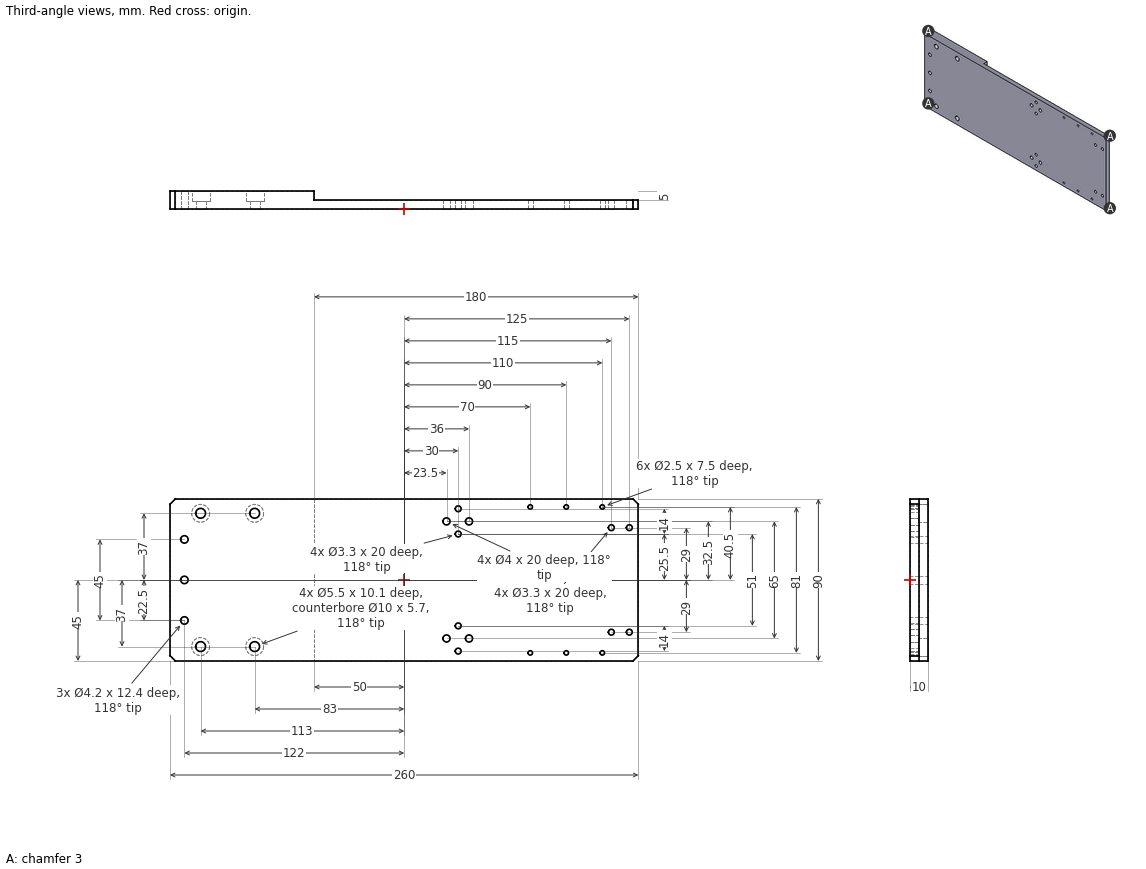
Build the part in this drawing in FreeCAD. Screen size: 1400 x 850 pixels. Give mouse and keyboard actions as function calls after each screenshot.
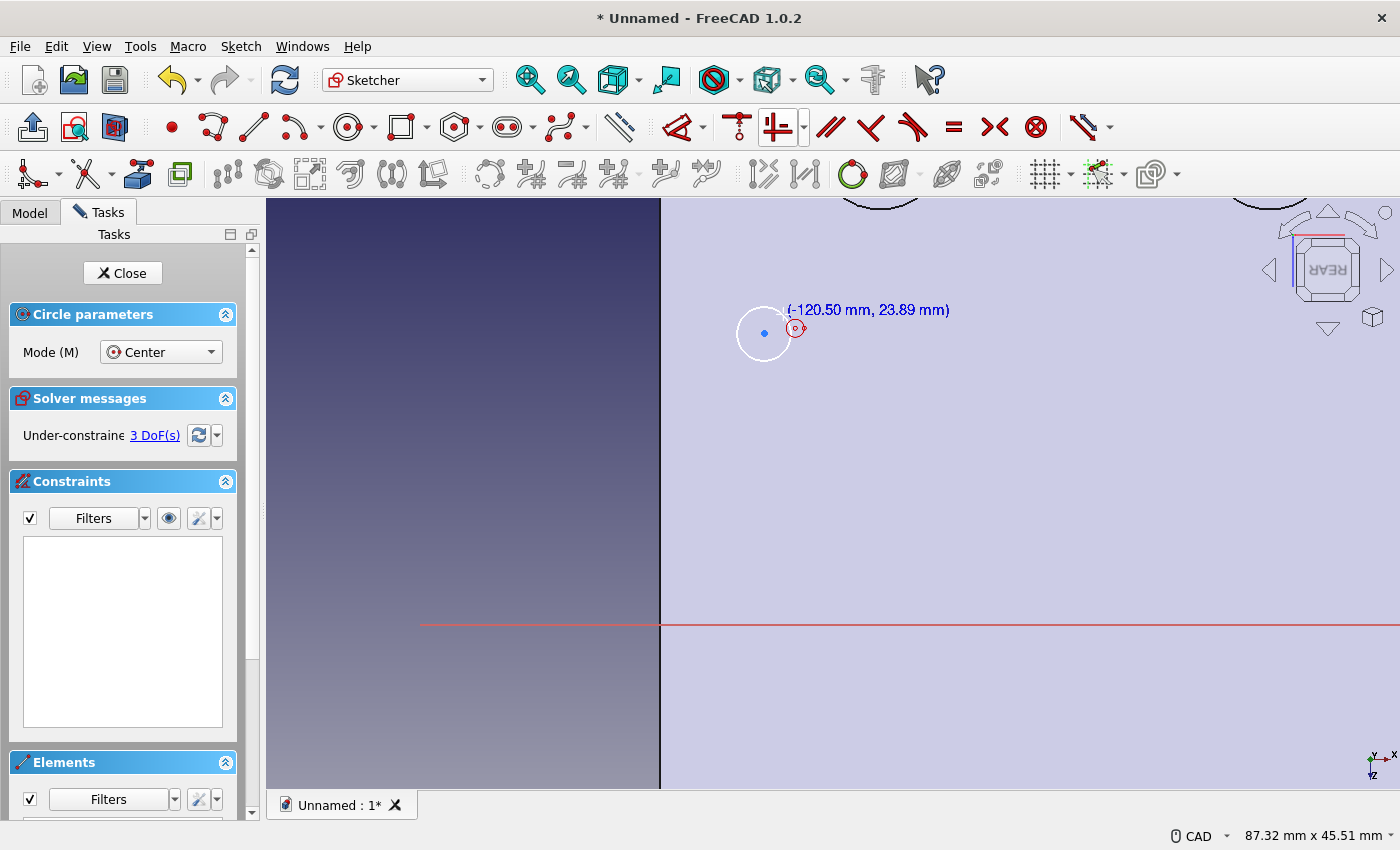
click(764, 625)
click(783, 606)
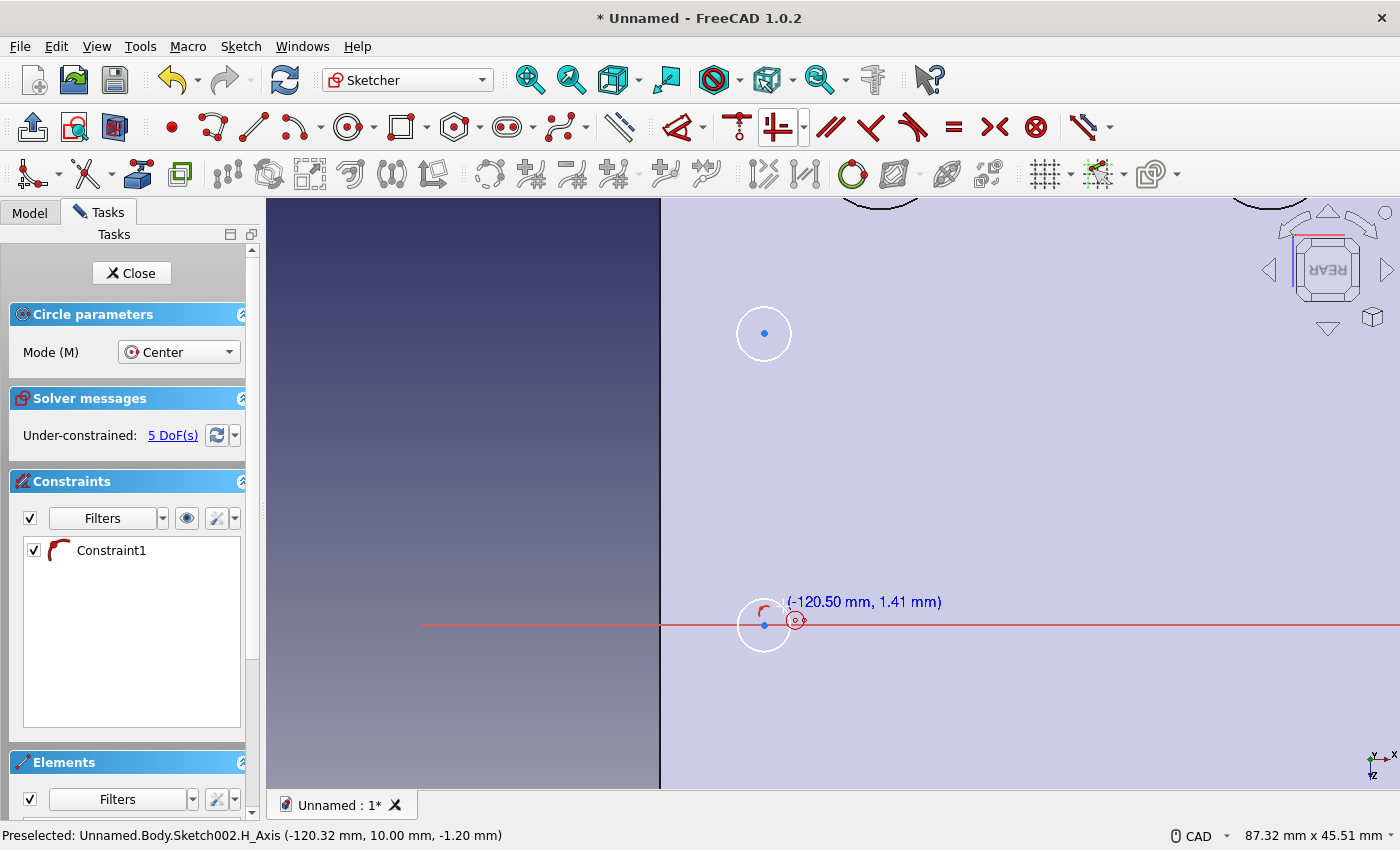
scroll(766, 333, down, 3)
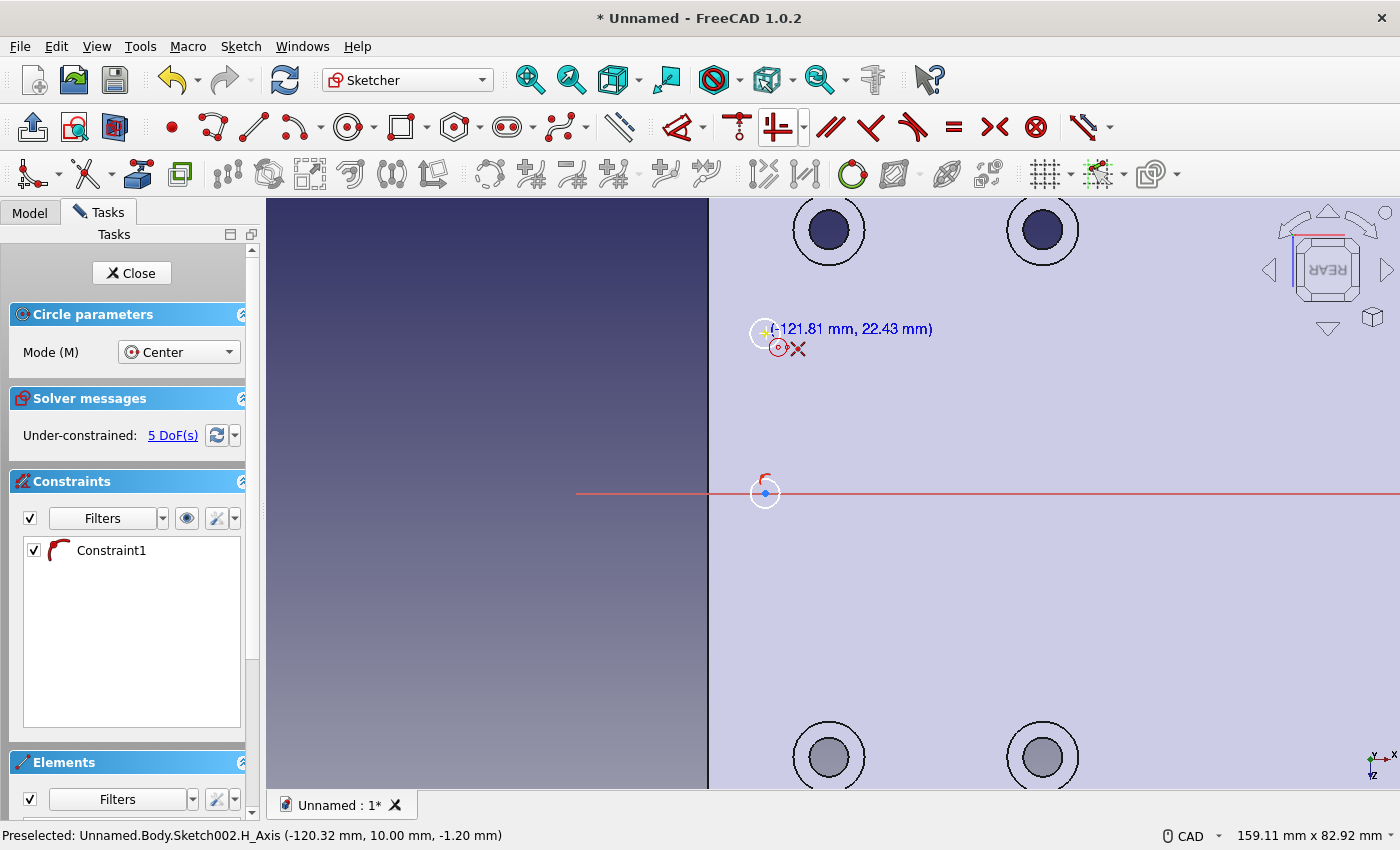
scroll(765, 654, up, 3)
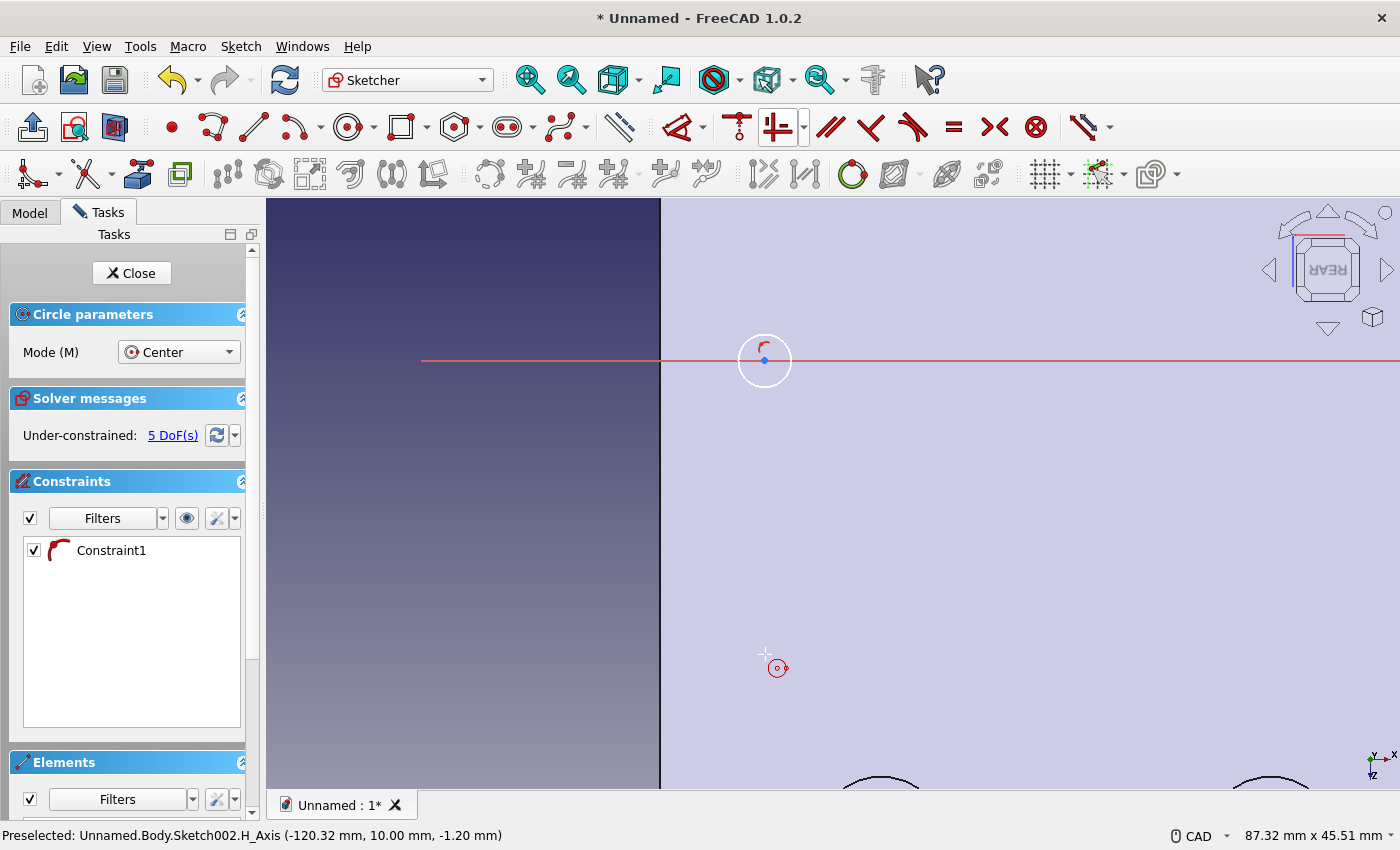
click(764, 653)
click(784, 634)
key(Escape)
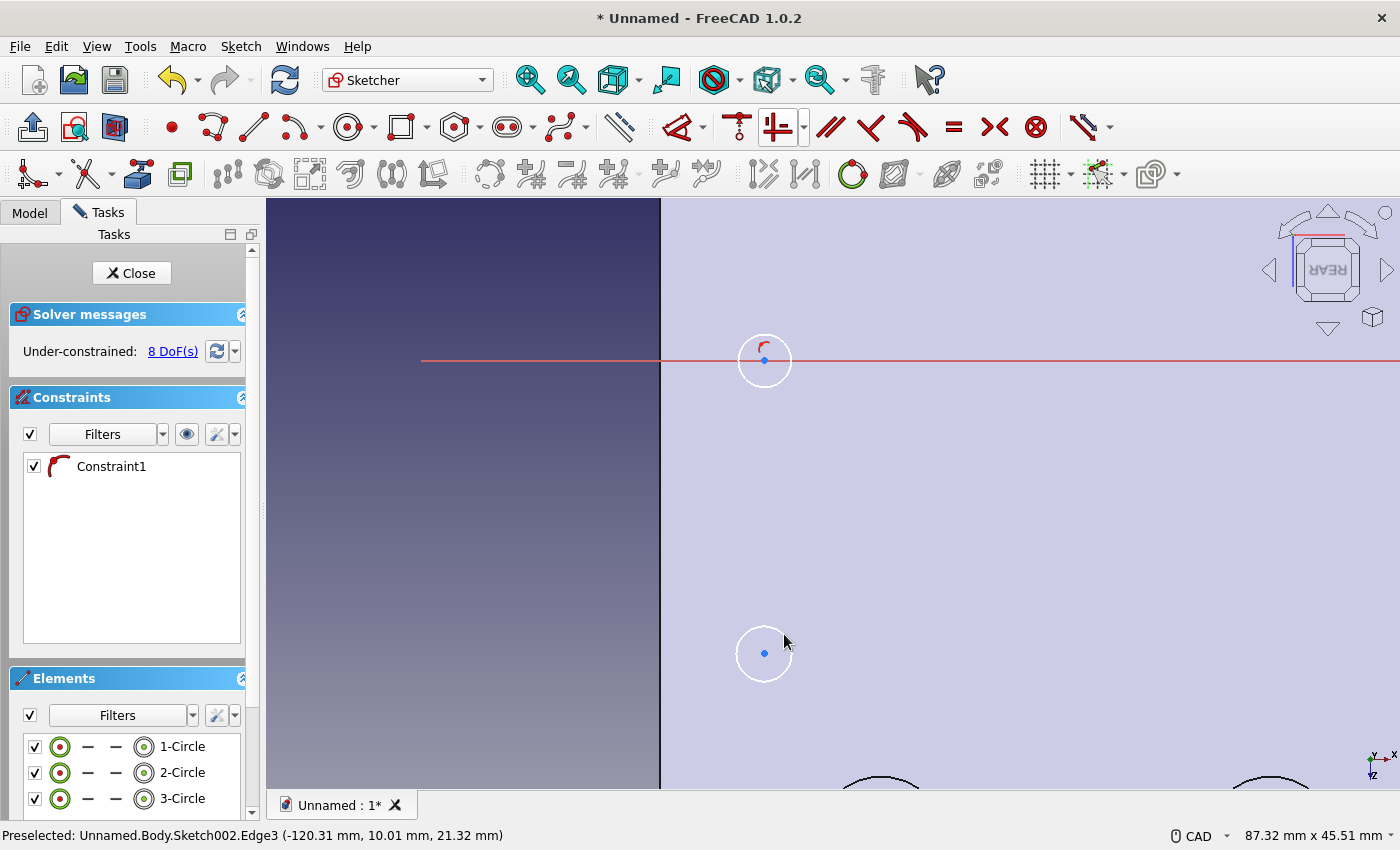
scroll(765, 655, down, 3)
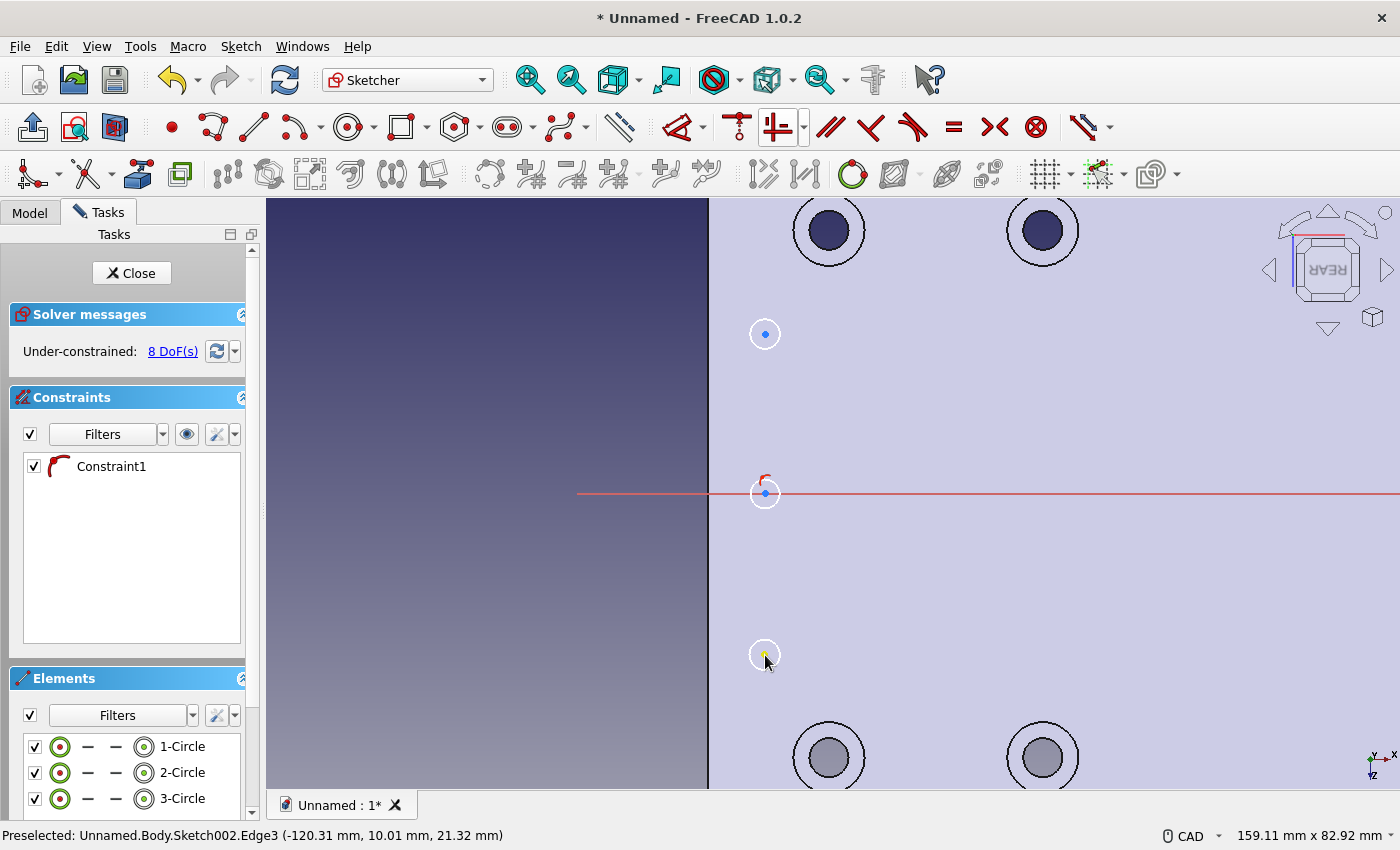
click(775, 324)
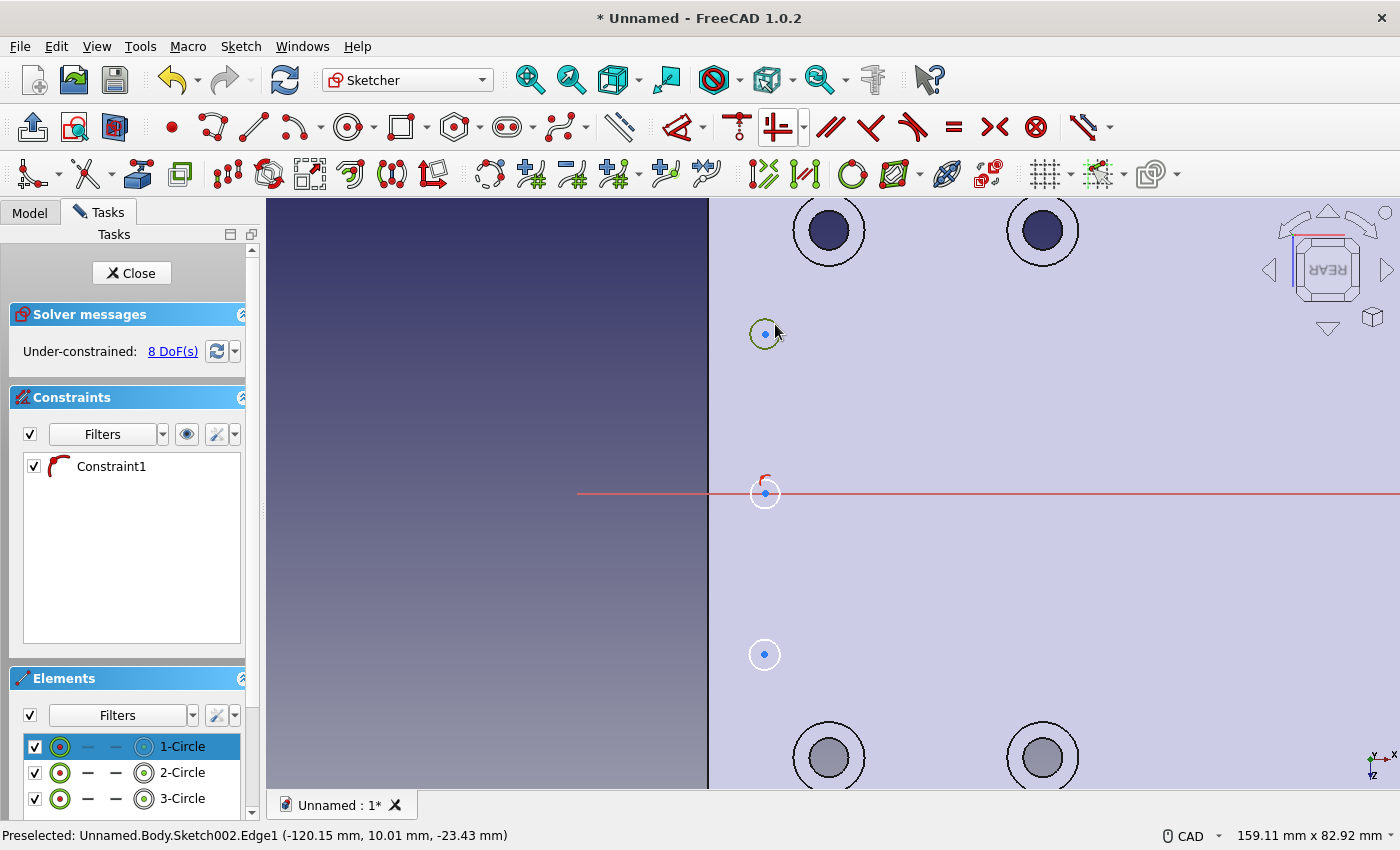
scroll(775, 484, up, 2)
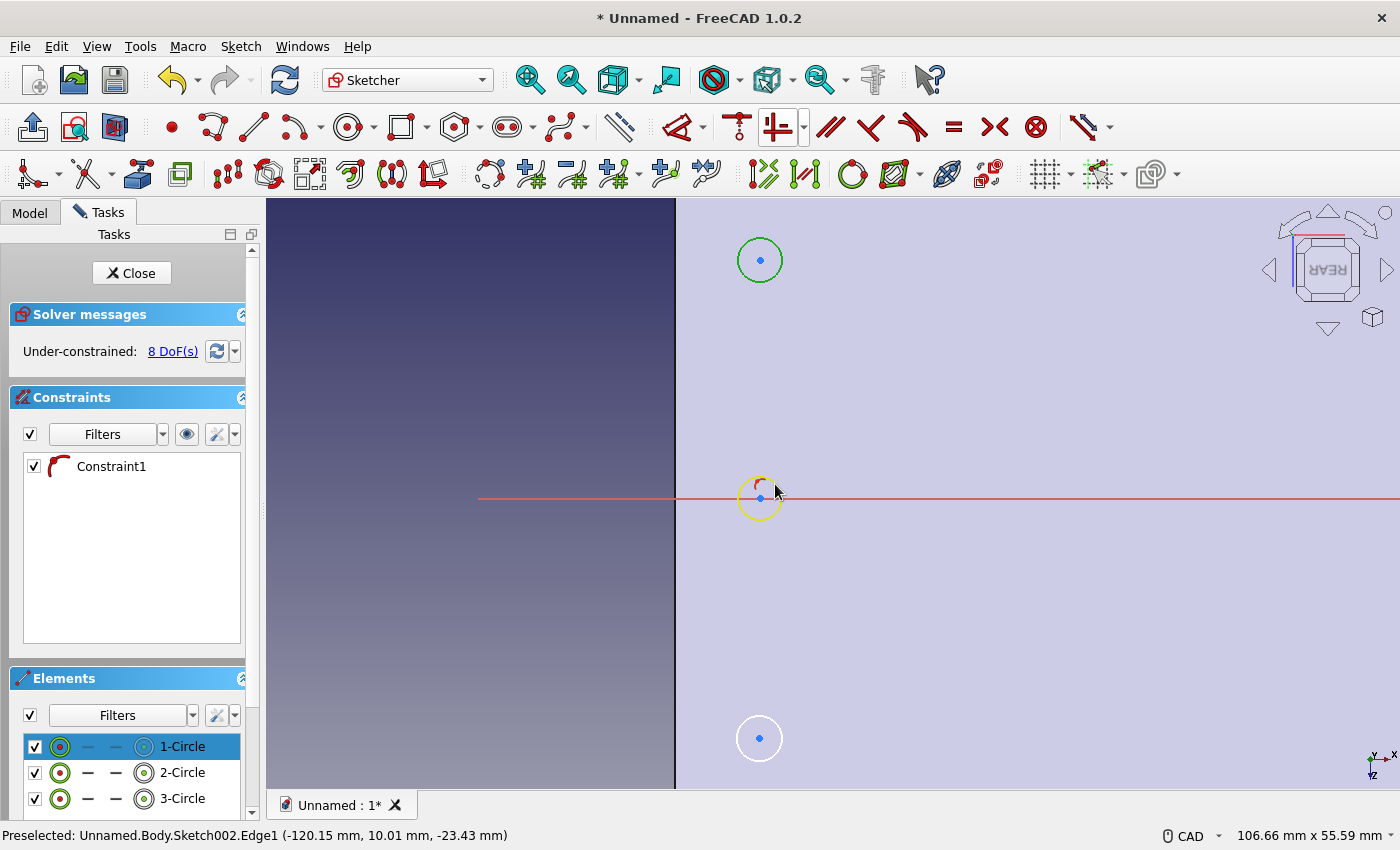
click(775, 483)